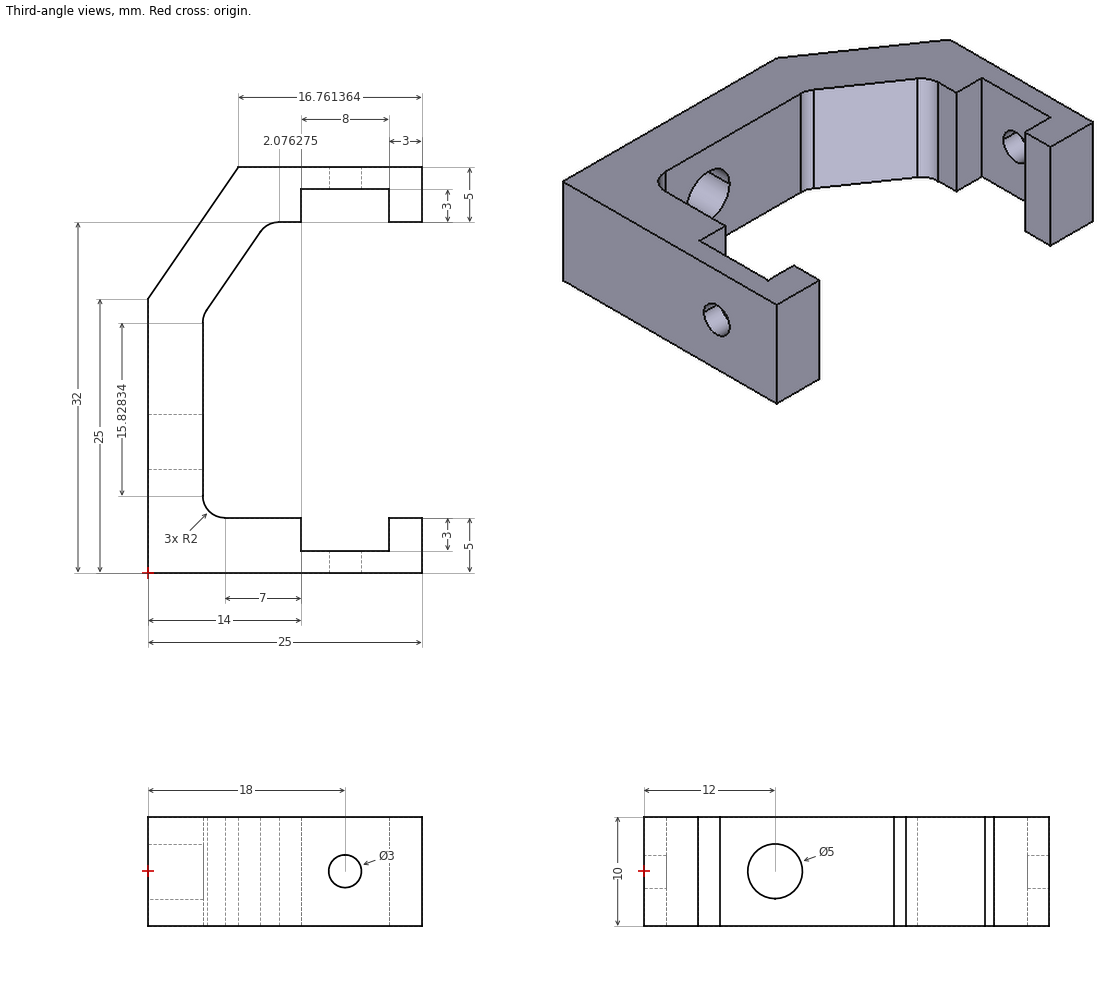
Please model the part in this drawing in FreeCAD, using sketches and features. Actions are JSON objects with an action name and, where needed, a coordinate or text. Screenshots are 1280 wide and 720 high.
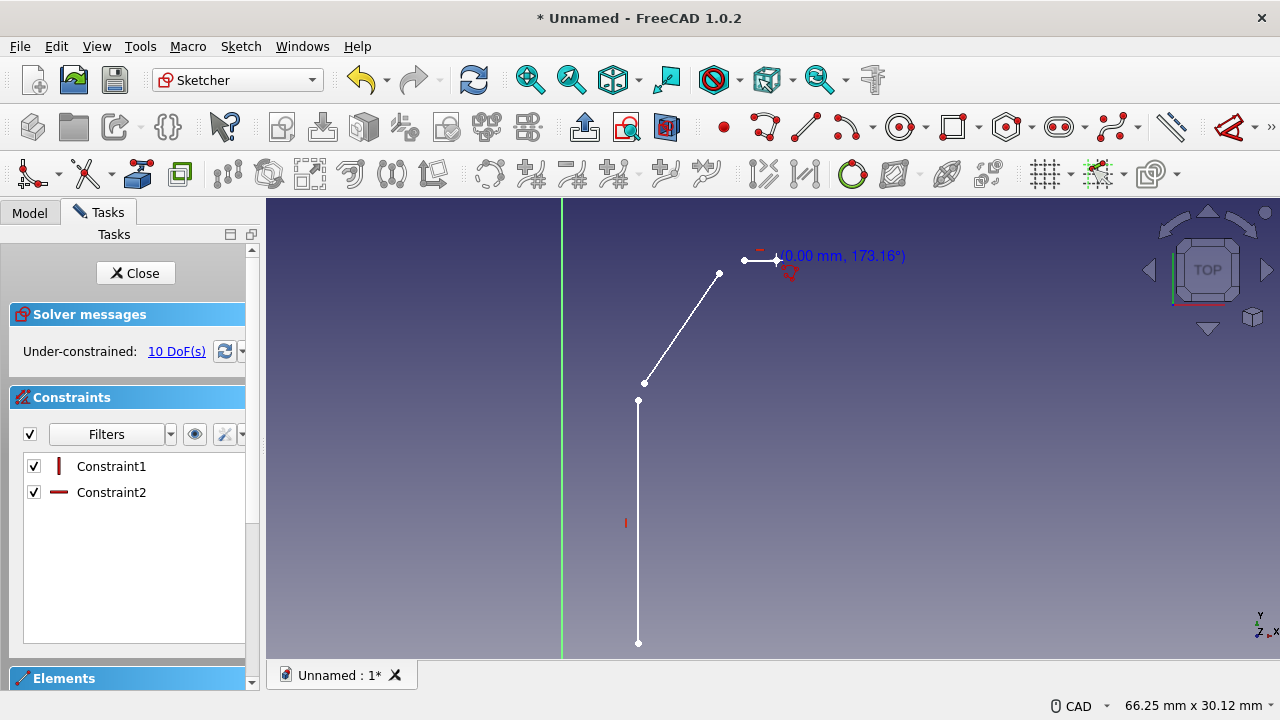
{"action": "scroll", "coordinate": [646, 383], "scroll_direction": "down", "scroll_amount": 3}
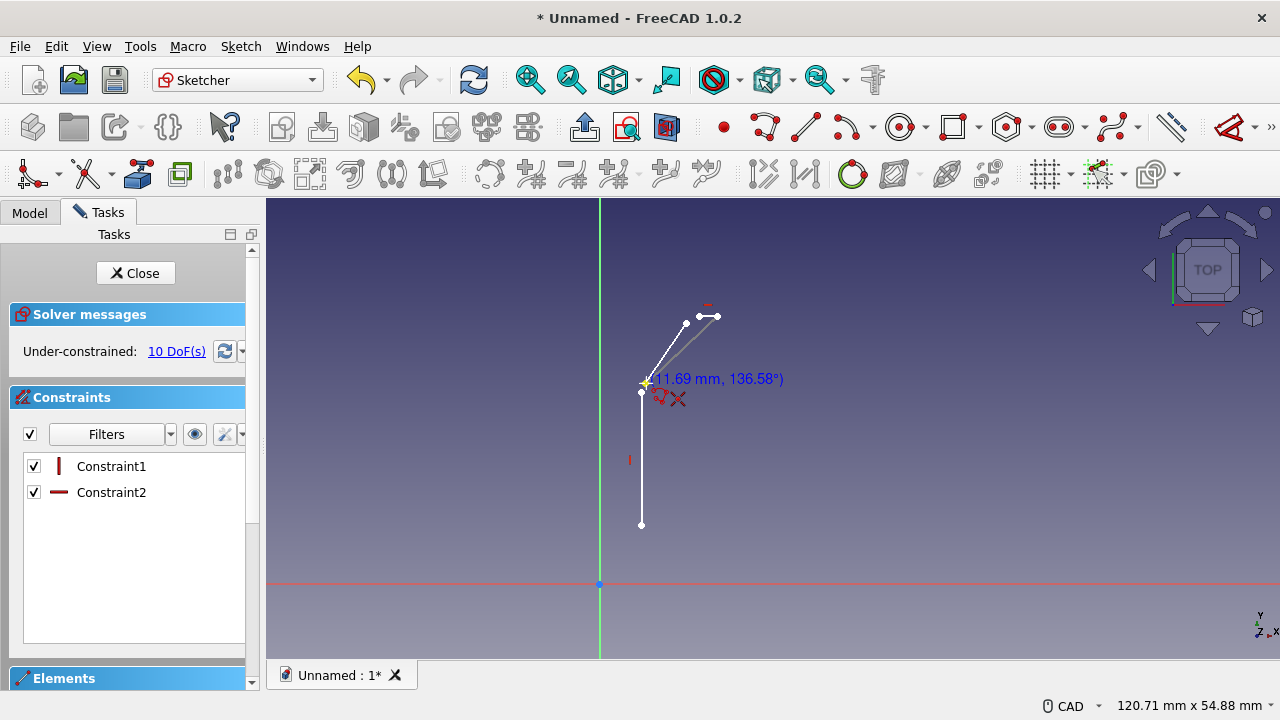
{"action": "left_click", "coordinate": [718, 290]}
{"action": "left_click", "coordinate": [785, 290]}
{"action": "left_click", "coordinate": [785, 315]}
{"action": "left_click", "coordinate": [810, 315]}
{"action": "left_click", "coordinate": [810, 273]}
{"action": "left_click", "coordinate": [669, 273]}
{"action": "left_click", "coordinate": [600, 374]}
{"action": "left_click", "coordinate": [600, 584]}
{"action": "left_click", "coordinate": [810, 575]}
{"action": "left_click", "coordinate": [810, 542]}
{"action": "left_click", "coordinate": [785, 542]}
{"action": "left_click", "coordinate": [785, 567]}
{"action": "left_click", "coordinate": [717, 567]}
{"action": "left_click", "coordinate": [717, 542]}
{"action": "left_click", "coordinate": [659, 542]}
{"action": "right_click", "coordinate": [659, 542]}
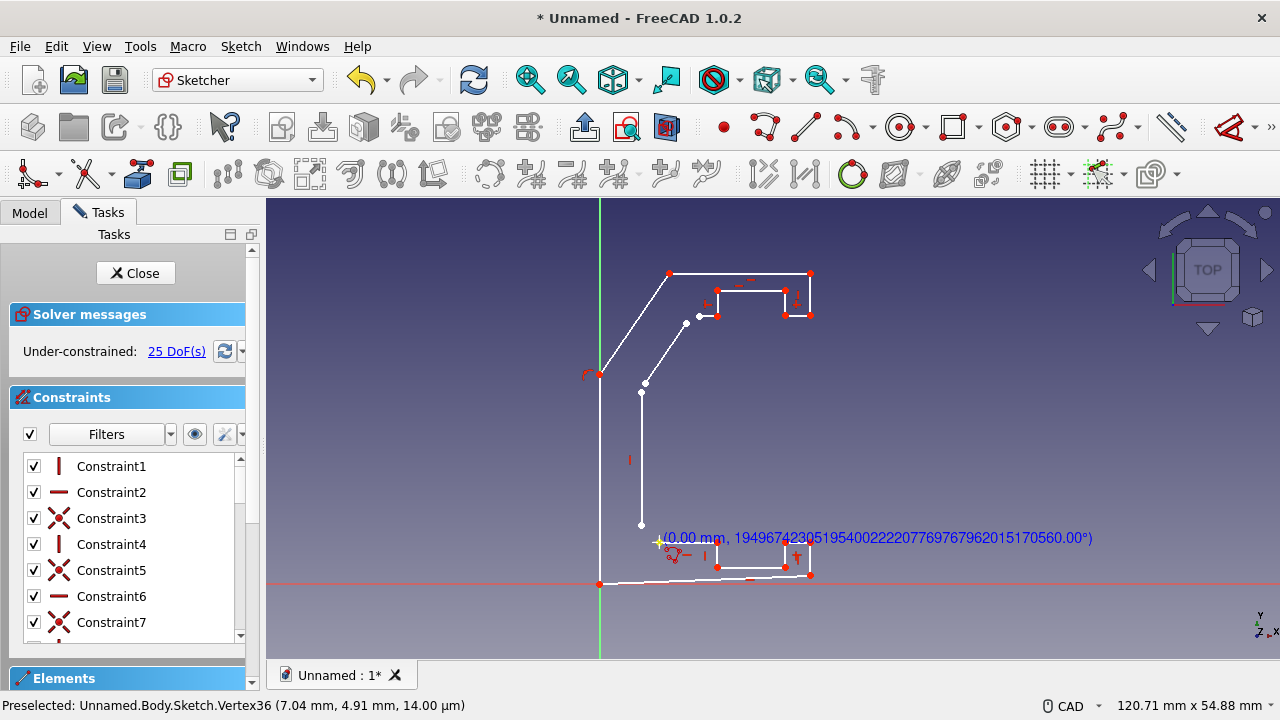
{"action": "left_click", "coordinate": [872, 128]}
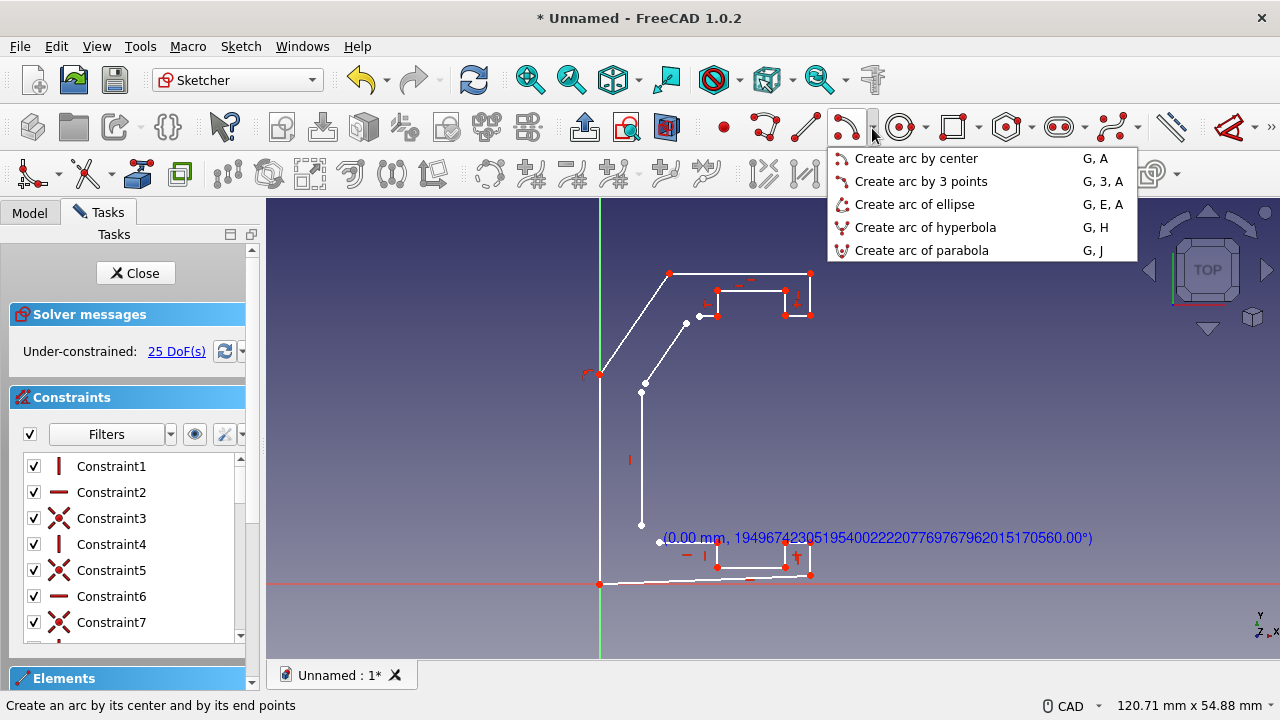
{"action": "left_click", "coordinate": [982, 182]}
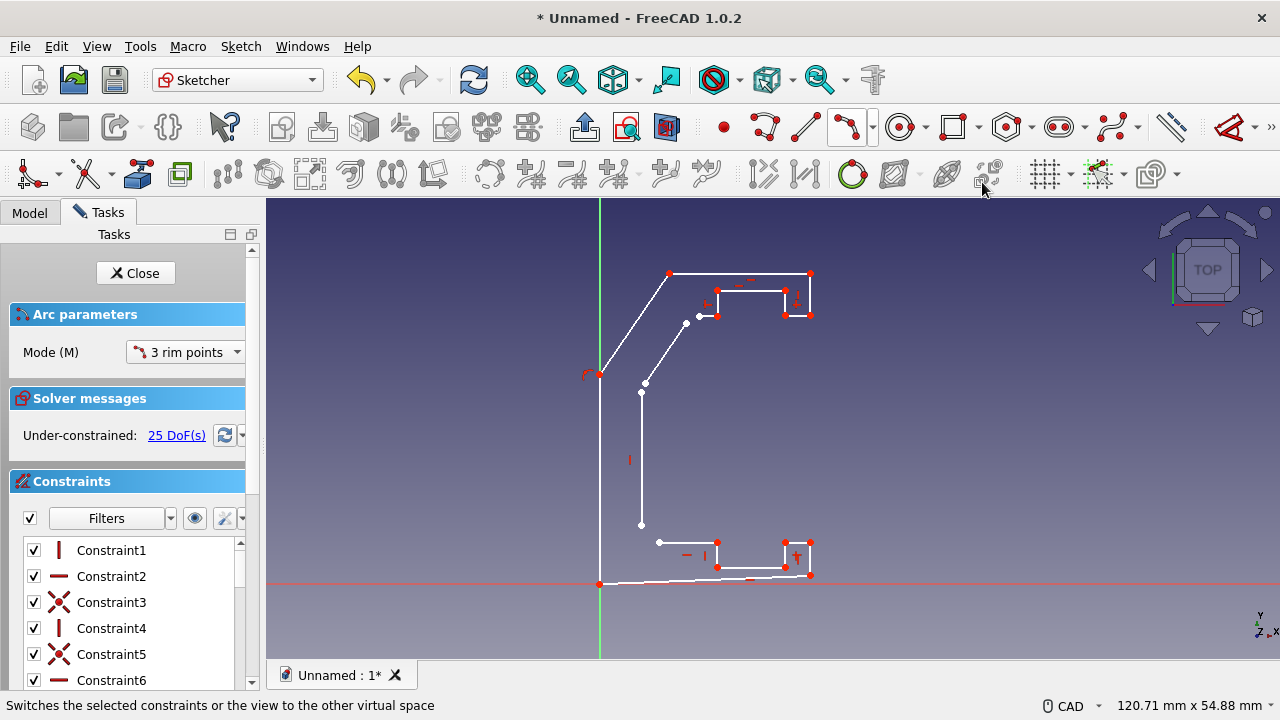
{"action": "scroll", "coordinate": [642, 392], "scroll_direction": "up", "scroll_amount": 3}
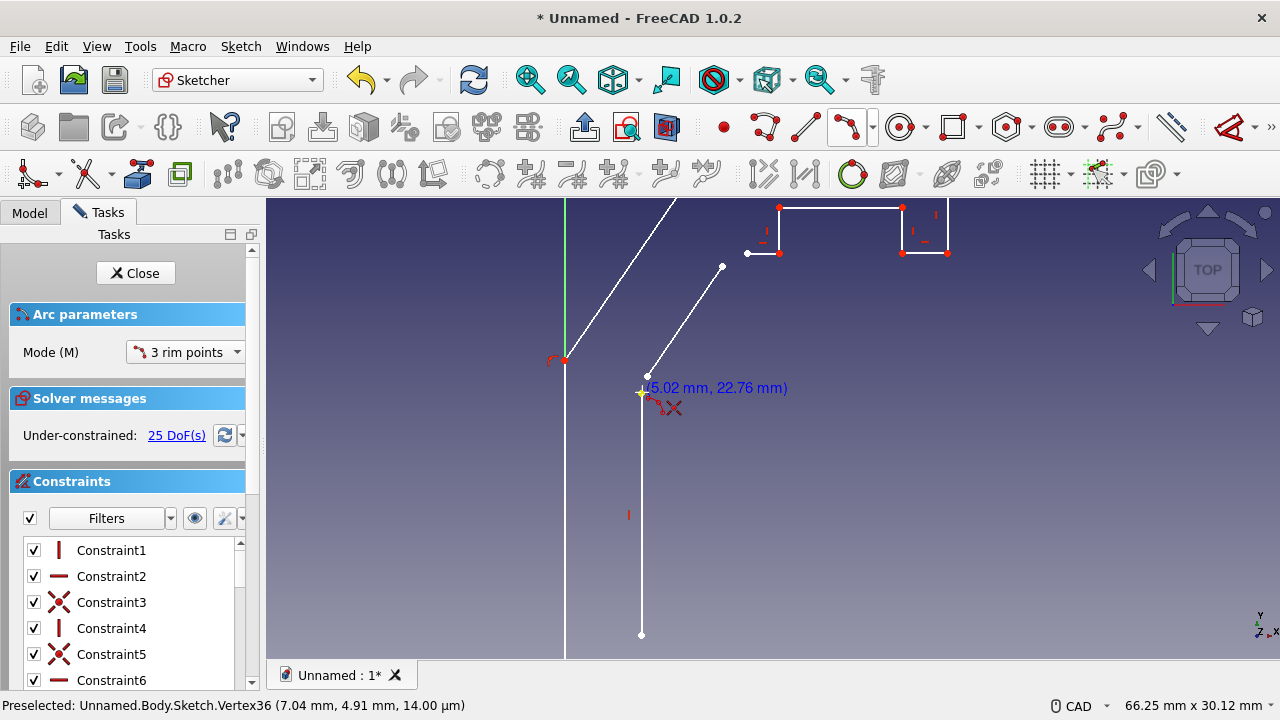
{"action": "left_click", "coordinate": [642, 393]}
{"action": "left_click", "coordinate": [647, 377]}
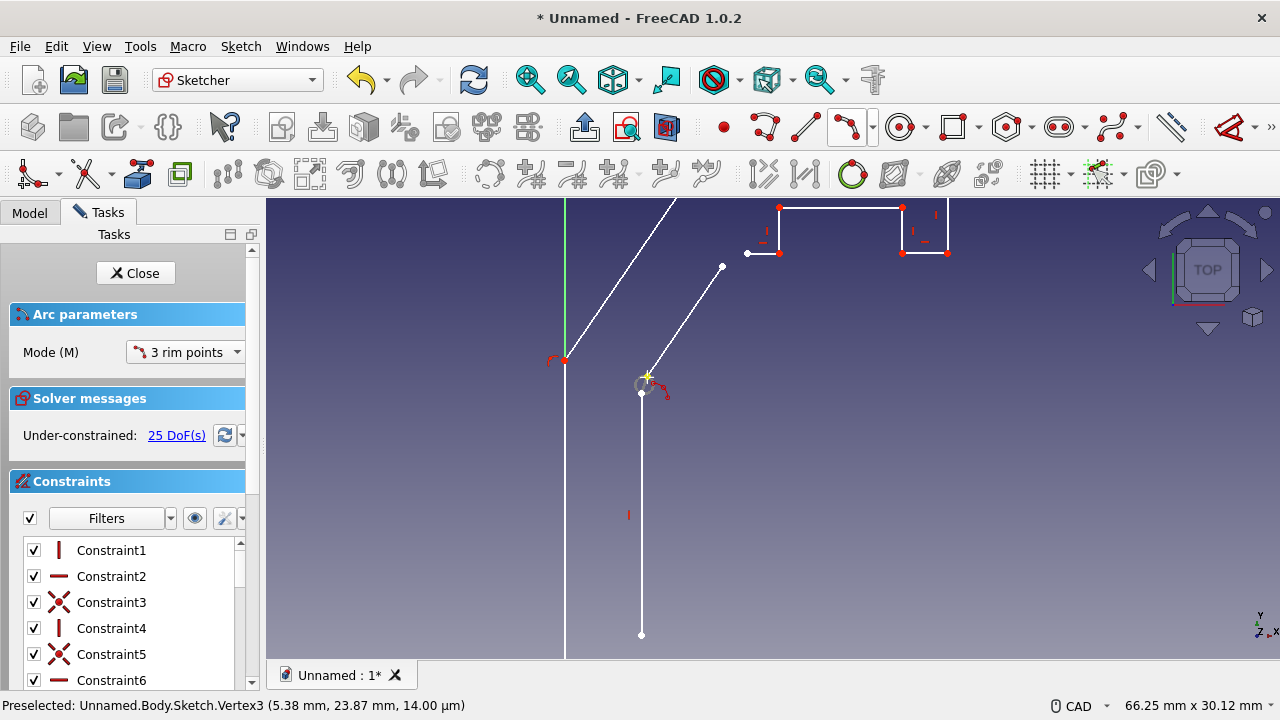
{"action": "scroll", "coordinate": [643, 383], "scroll_direction": "up", "scroll_amount": 13}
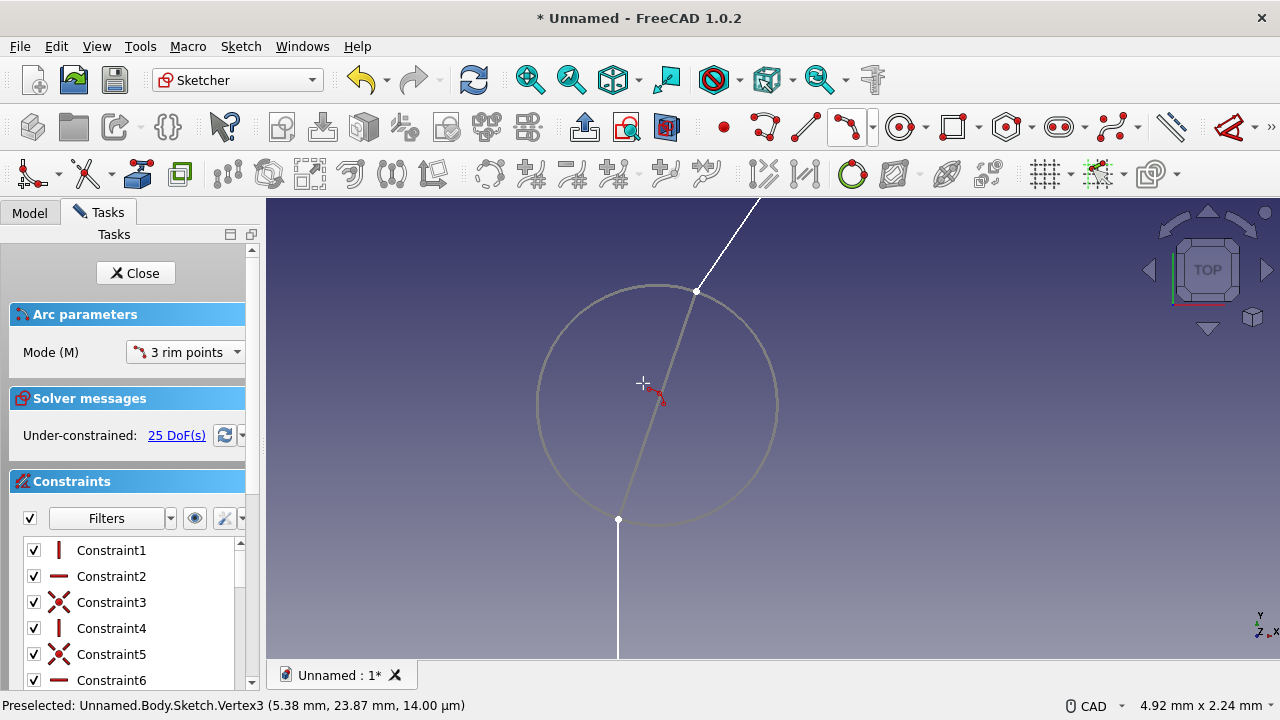
{"action": "left_click", "coordinate": [636, 384]}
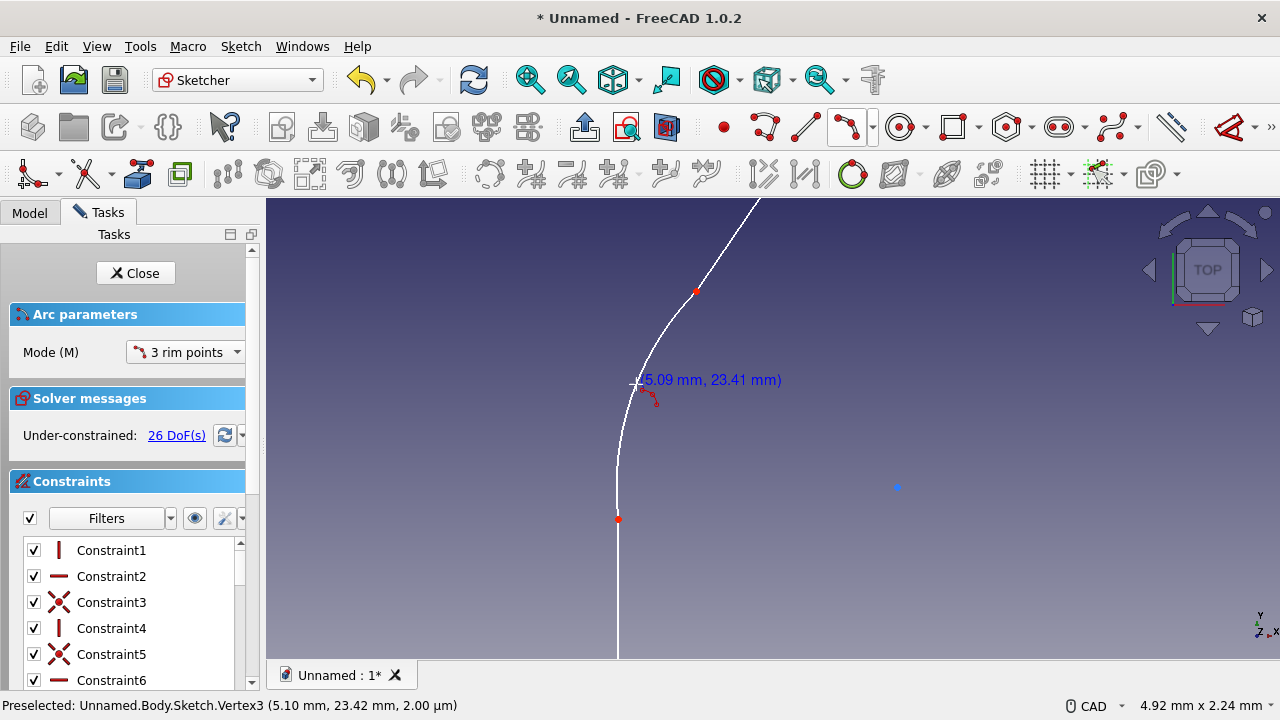
{"action": "scroll", "coordinate": [643, 387], "scroll_direction": "down", "scroll_amount": 16}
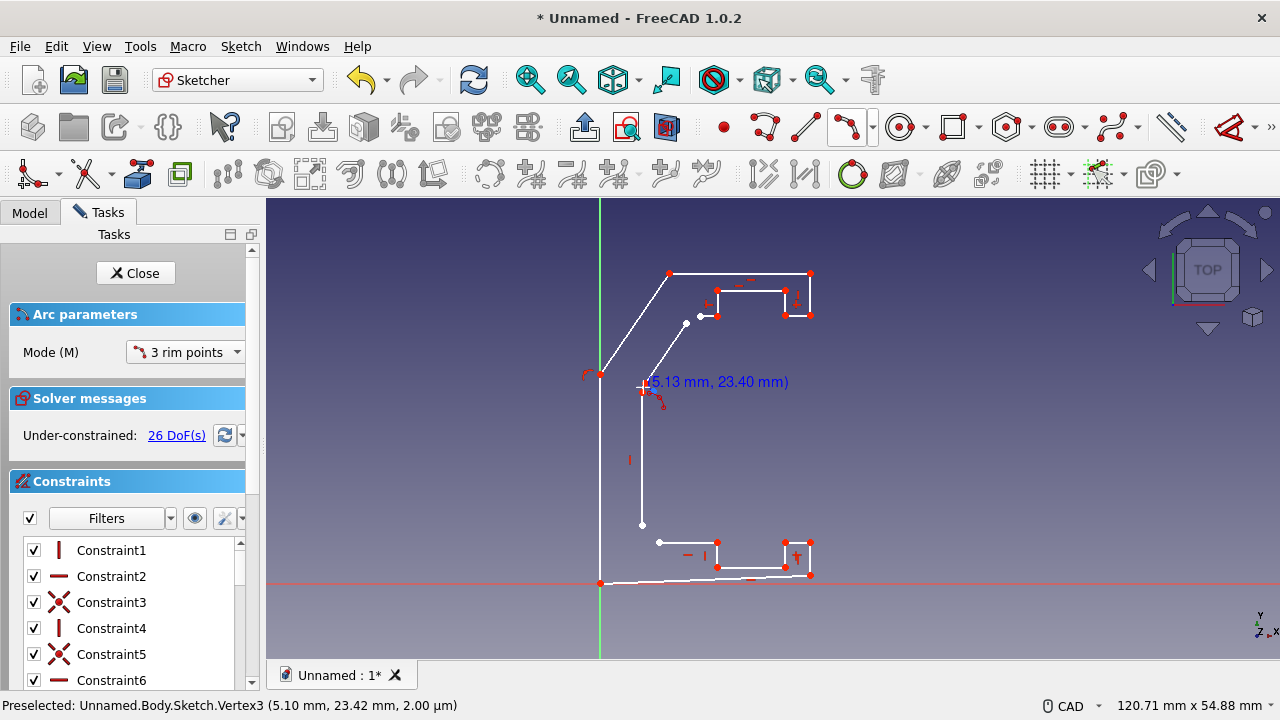
{"action": "left_click", "coordinate": [687, 323]}